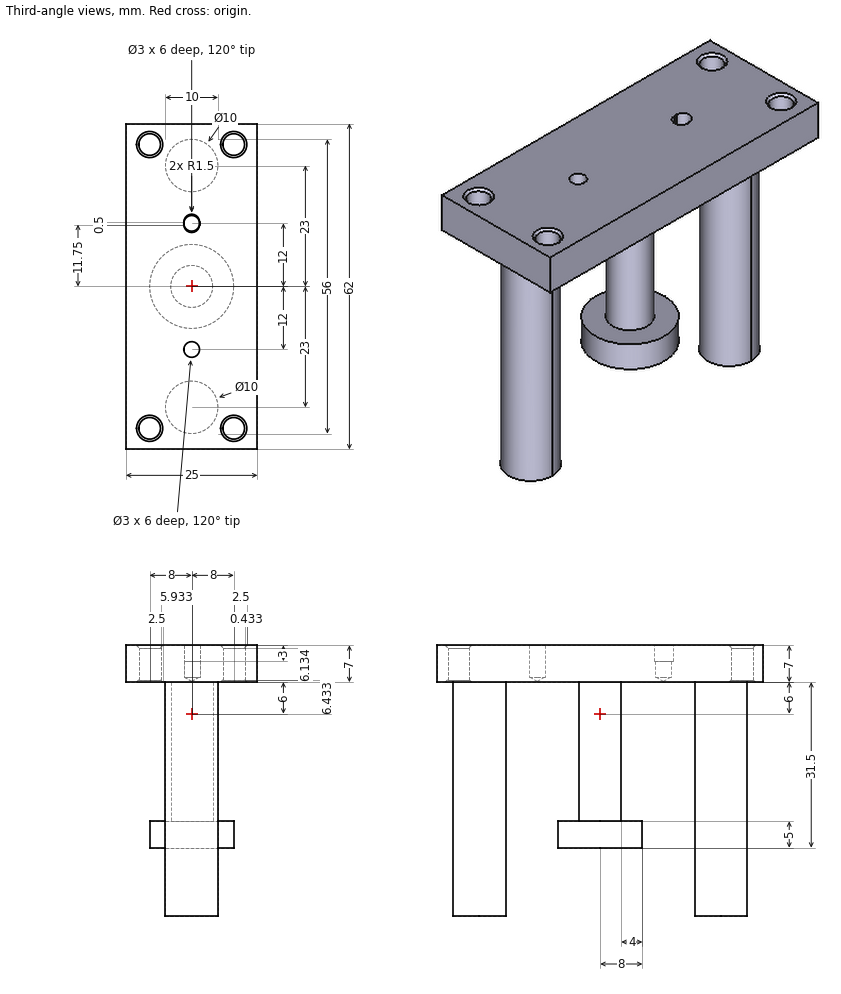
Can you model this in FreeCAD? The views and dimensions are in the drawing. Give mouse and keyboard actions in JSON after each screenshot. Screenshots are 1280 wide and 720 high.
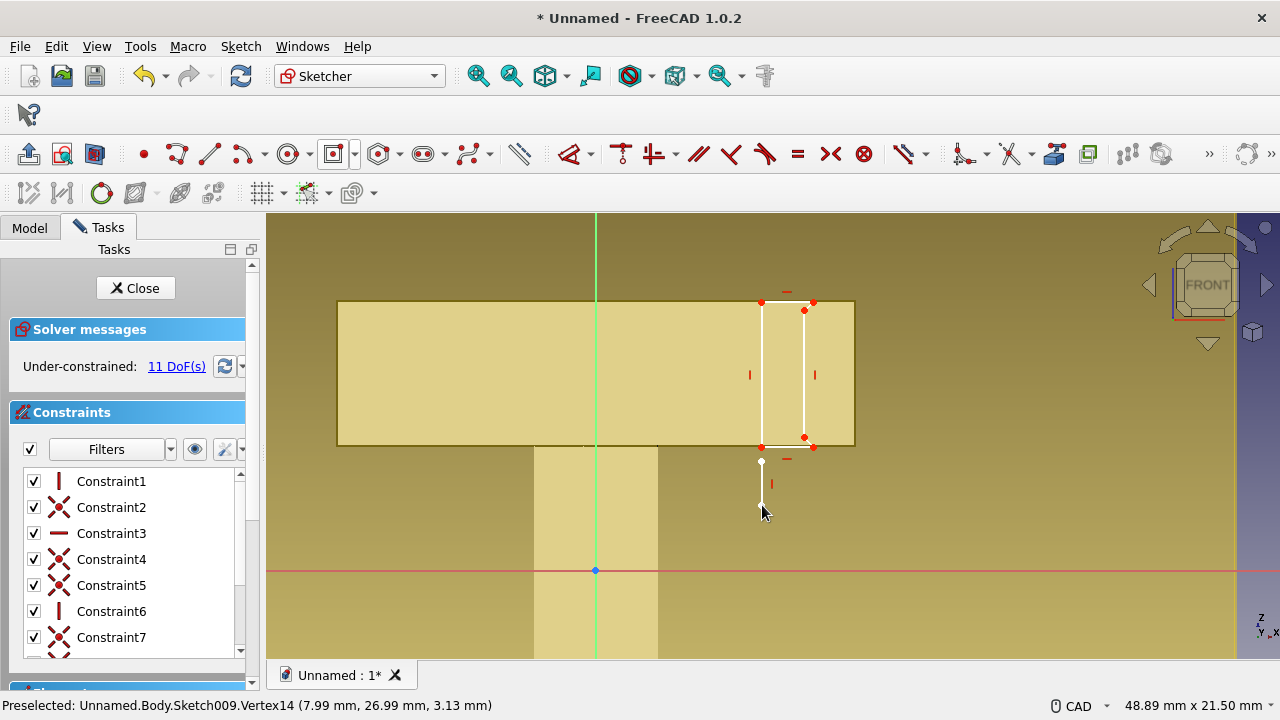
{"action": "left_click", "coordinate": [762, 475]}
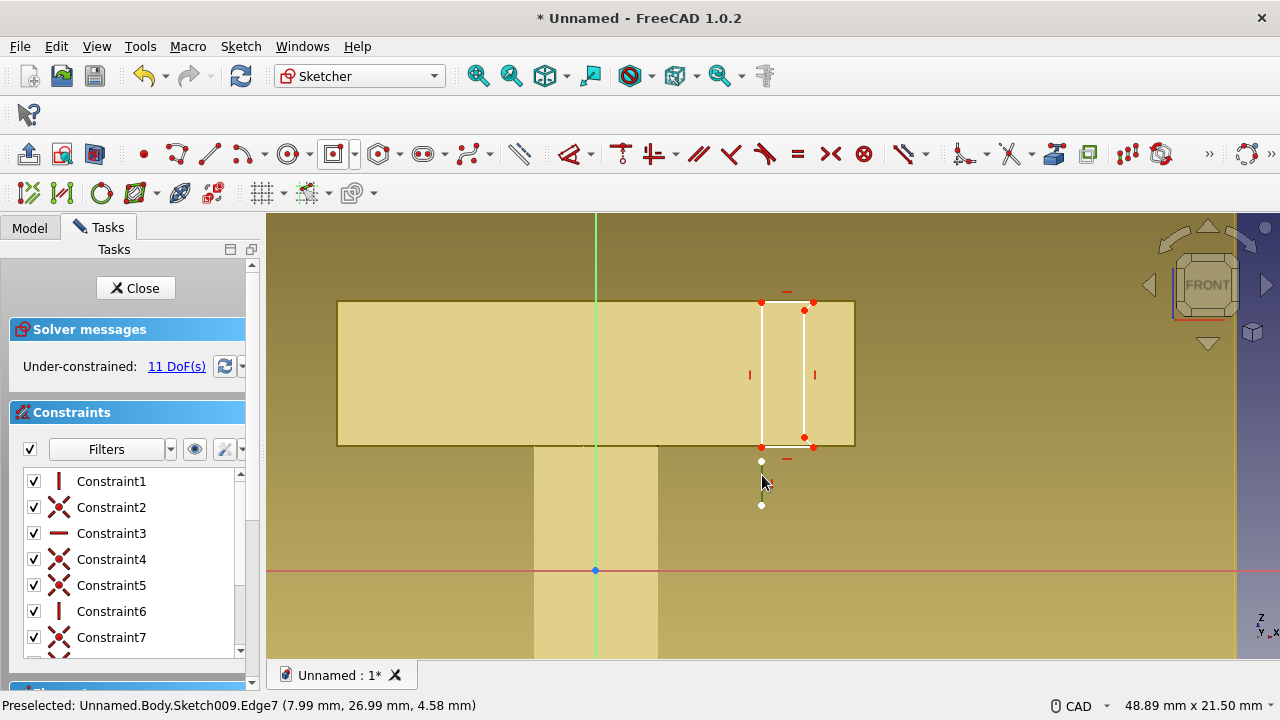
{"action": "left_click", "coordinate": [520, 154]}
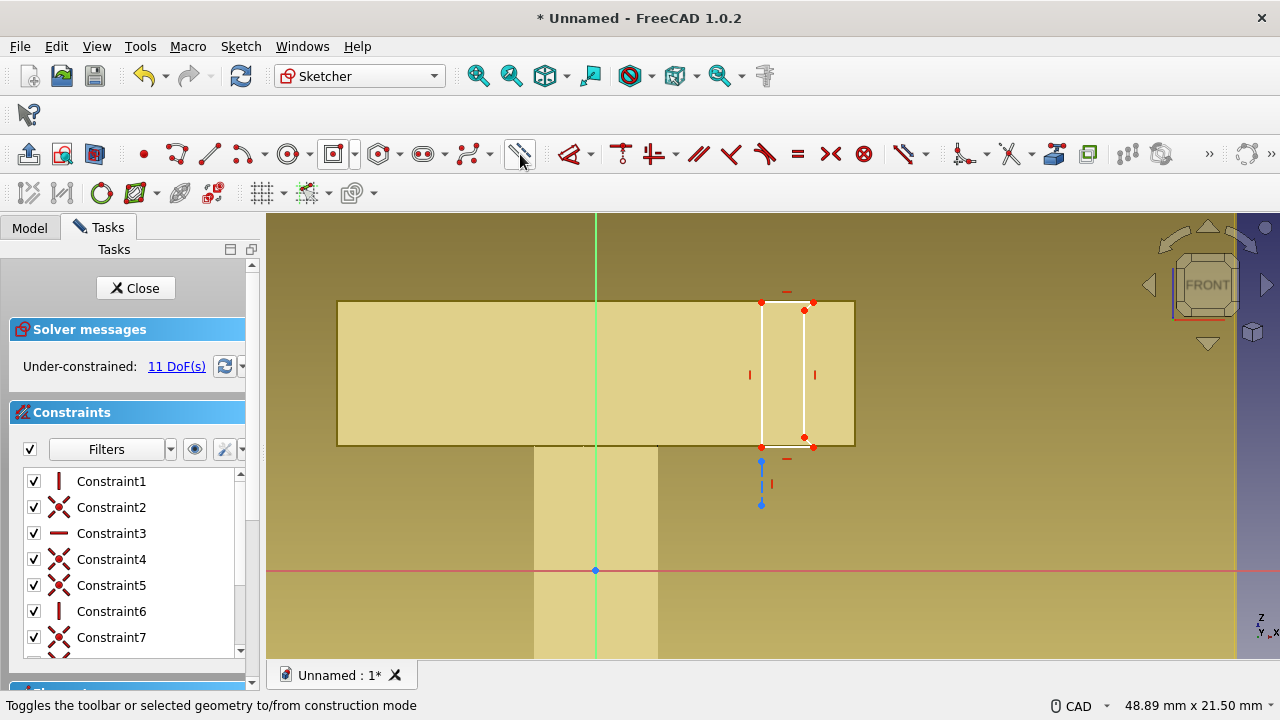
{"action": "left_click", "coordinate": [568, 154]}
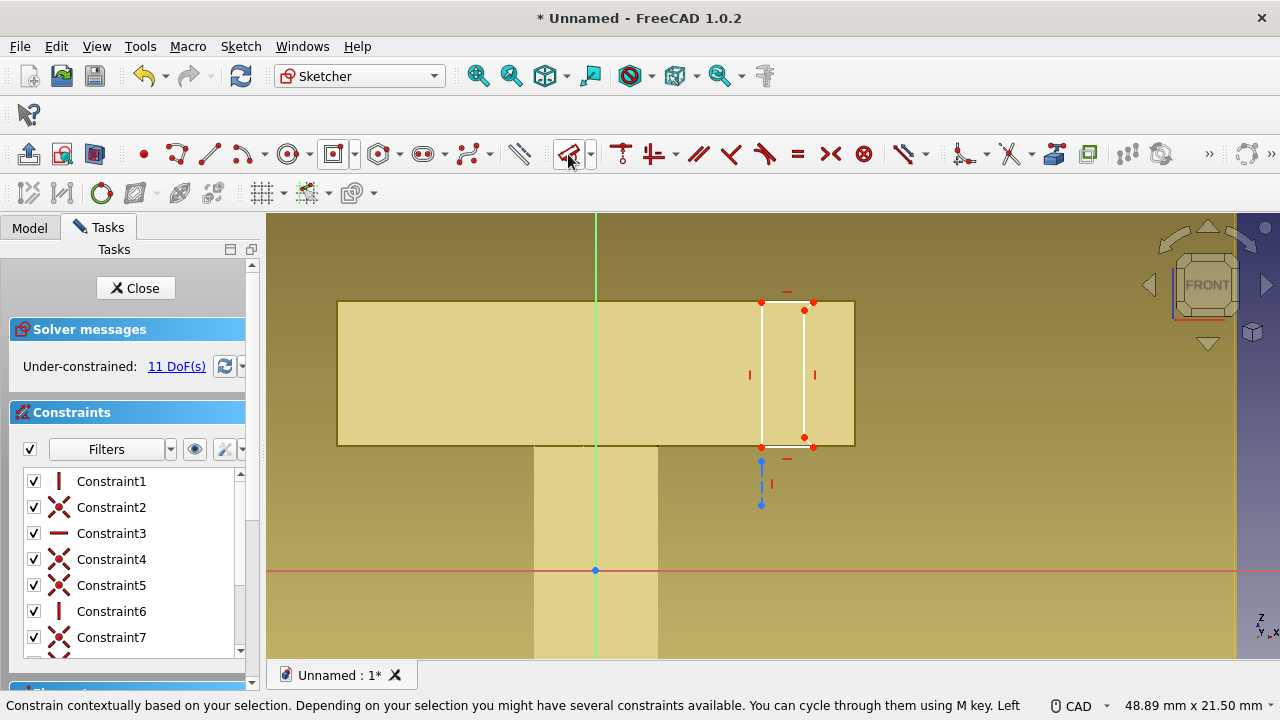
{"action": "left_click", "coordinate": [762, 404]}
{"action": "left_click", "coordinate": [728, 375]}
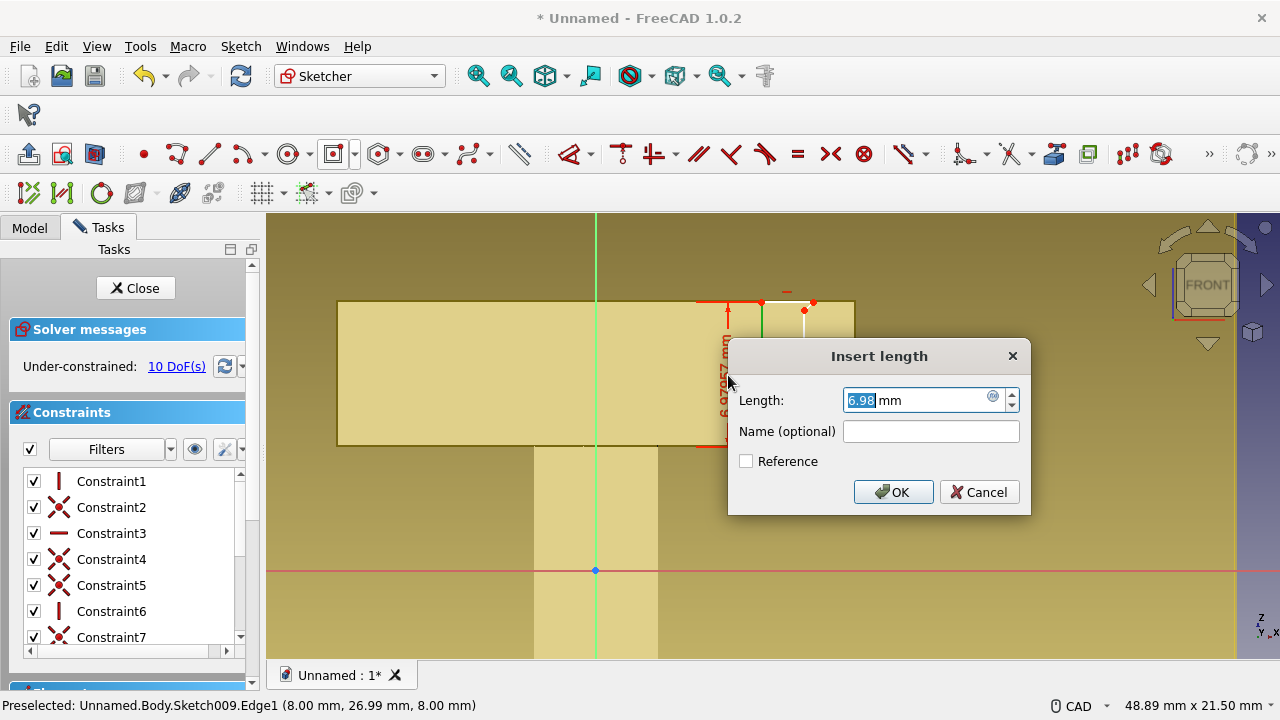
{"action": "type", "text": "7"}
{"action": "key", "text": "Return"}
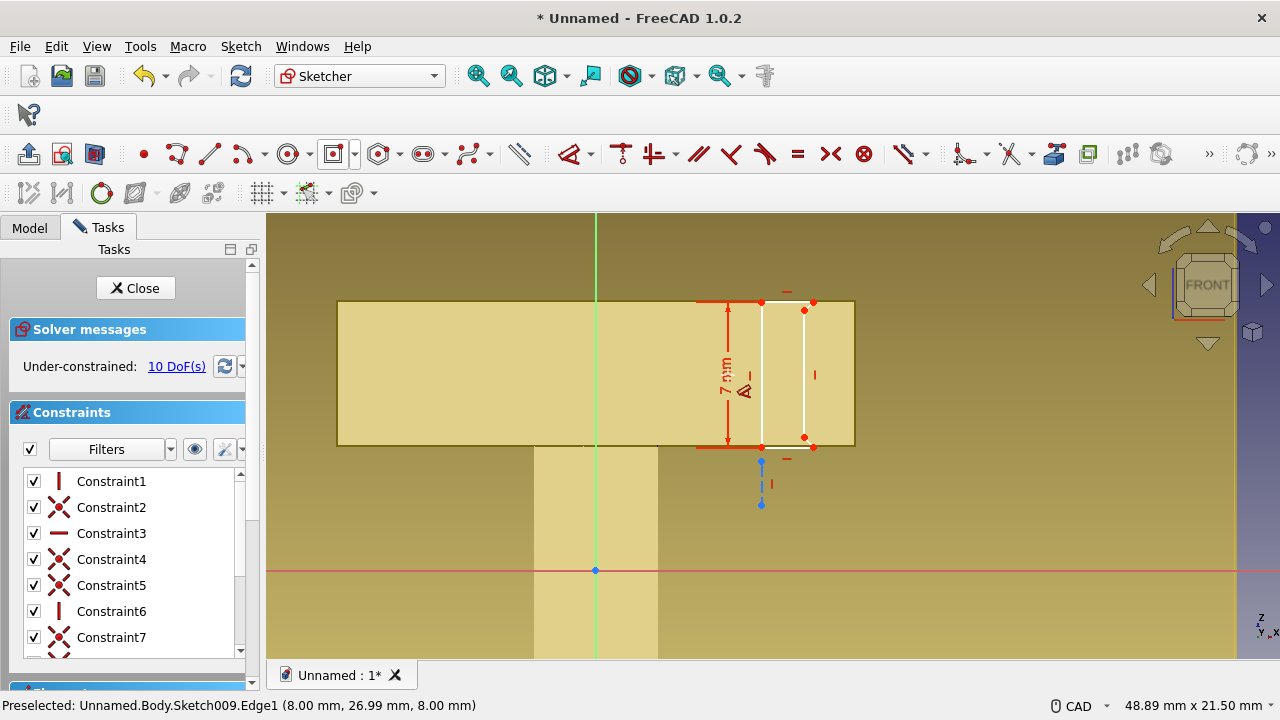
{"action": "left_click", "coordinate": [762, 448]}
{"action": "left_click", "coordinate": [679, 605]}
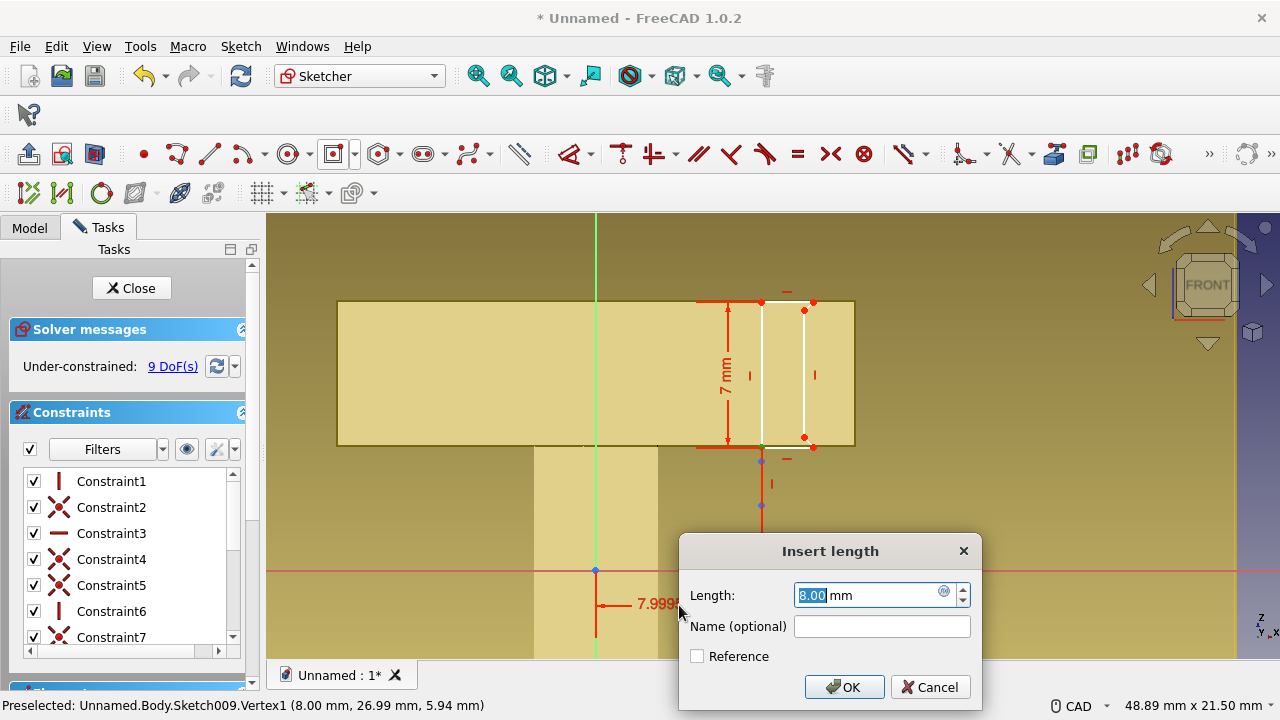
{"action": "type", "text": "8"}
{"action": "key", "text": "Return"}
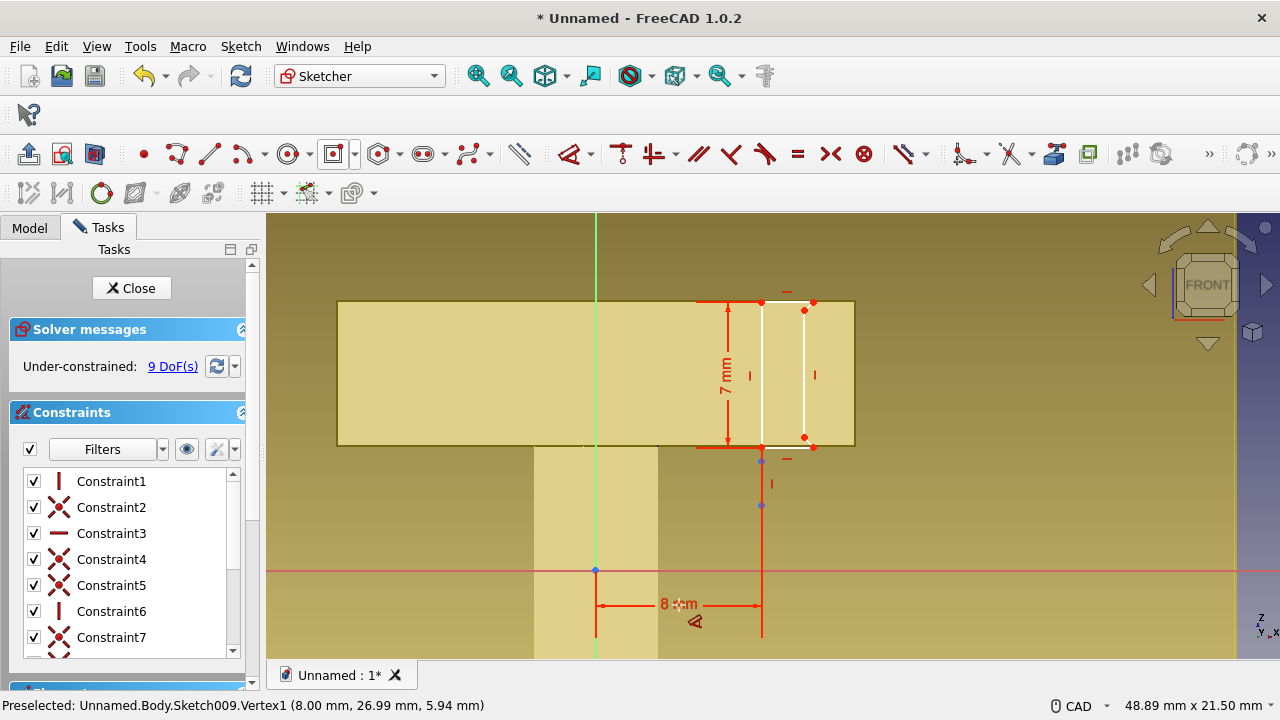
{"action": "left_click", "coordinate": [762, 448]}
{"action": "left_click", "coordinate": [562, 509]}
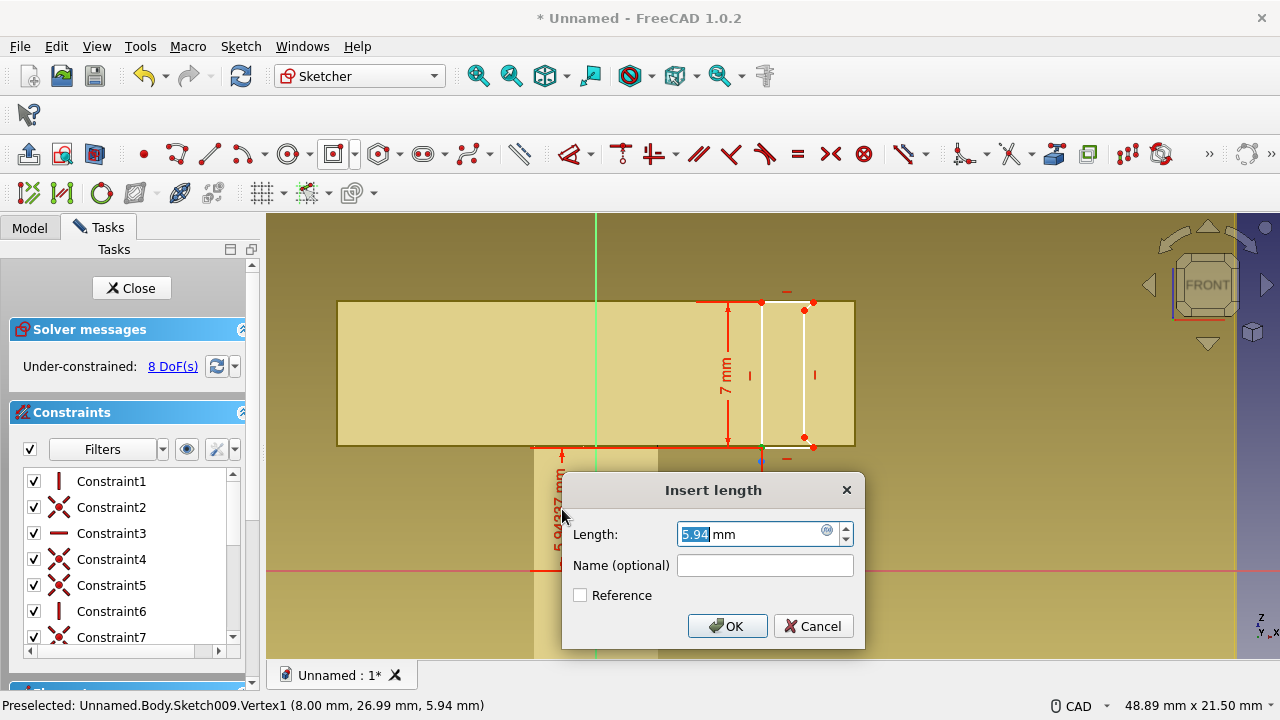
{"action": "type", "text": "6"}
{"action": "key", "text": "Return"}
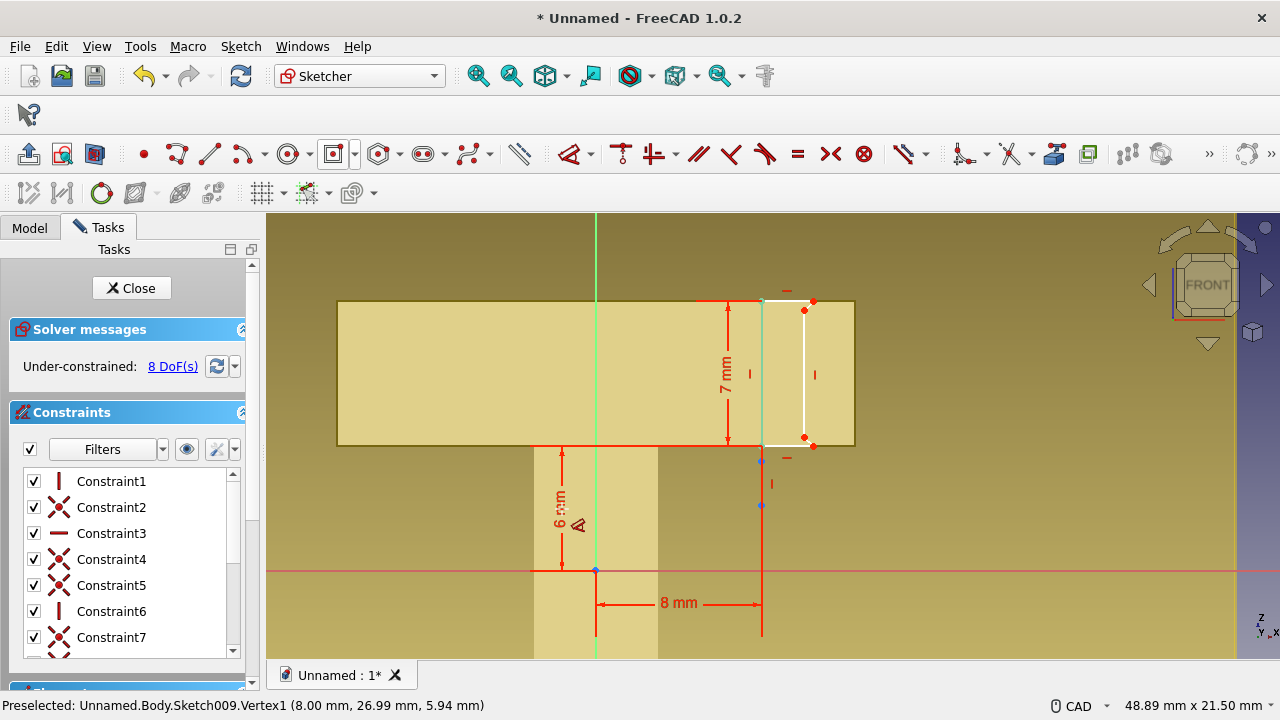
{"action": "left_click", "coordinate": [762, 461]}
{"action": "left_click", "coordinate": [679, 427]}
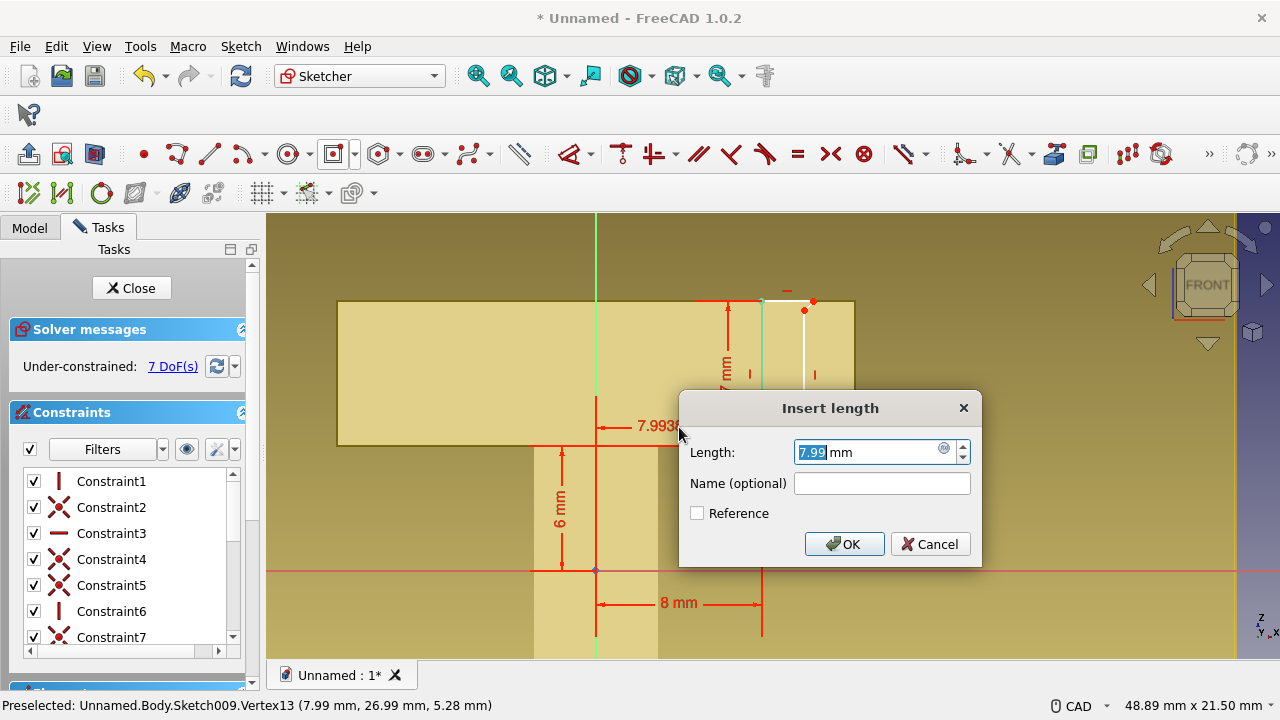
{"action": "type", "text": "8"}
{"action": "key", "text": "Return"}